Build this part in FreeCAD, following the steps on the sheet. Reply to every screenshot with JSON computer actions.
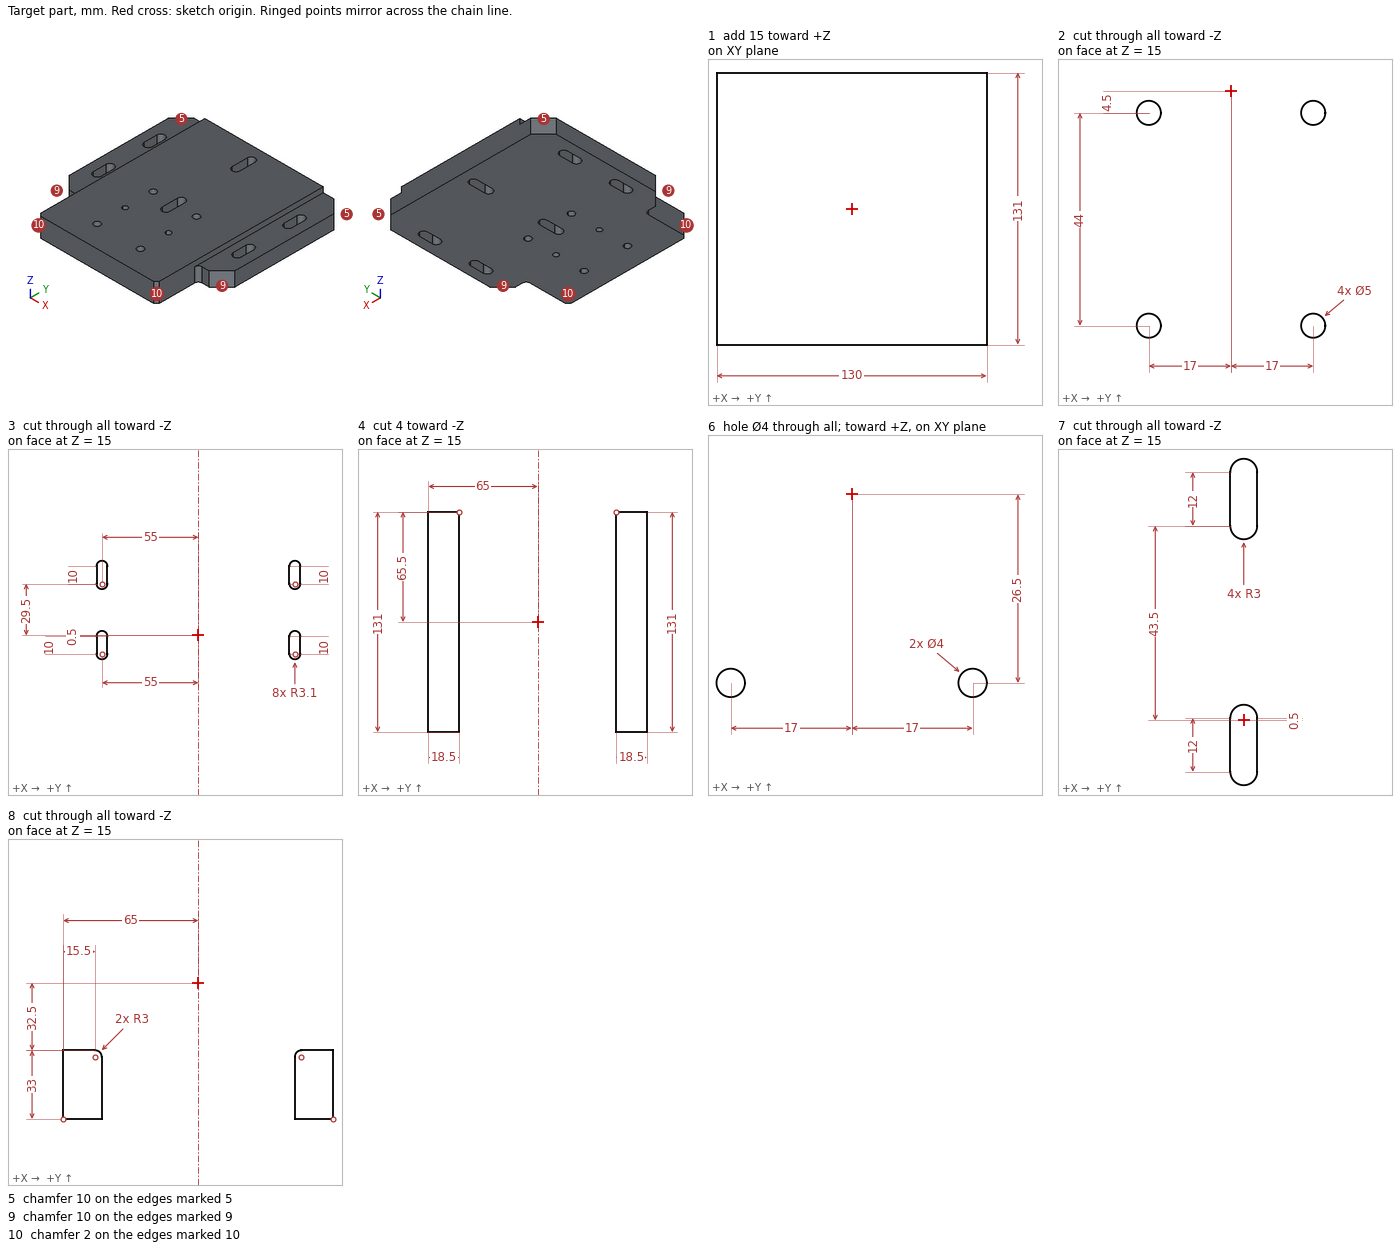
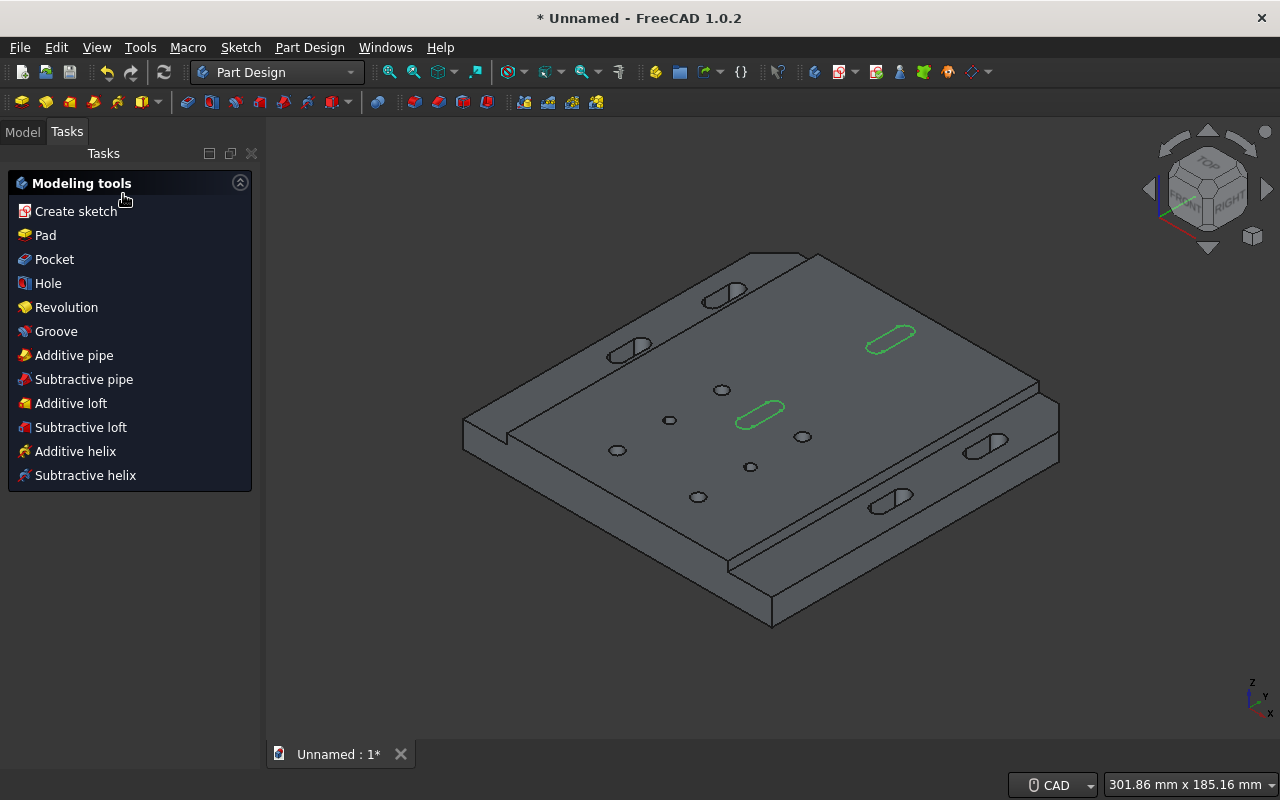
{"action": "left_click", "coordinate": [188, 102]}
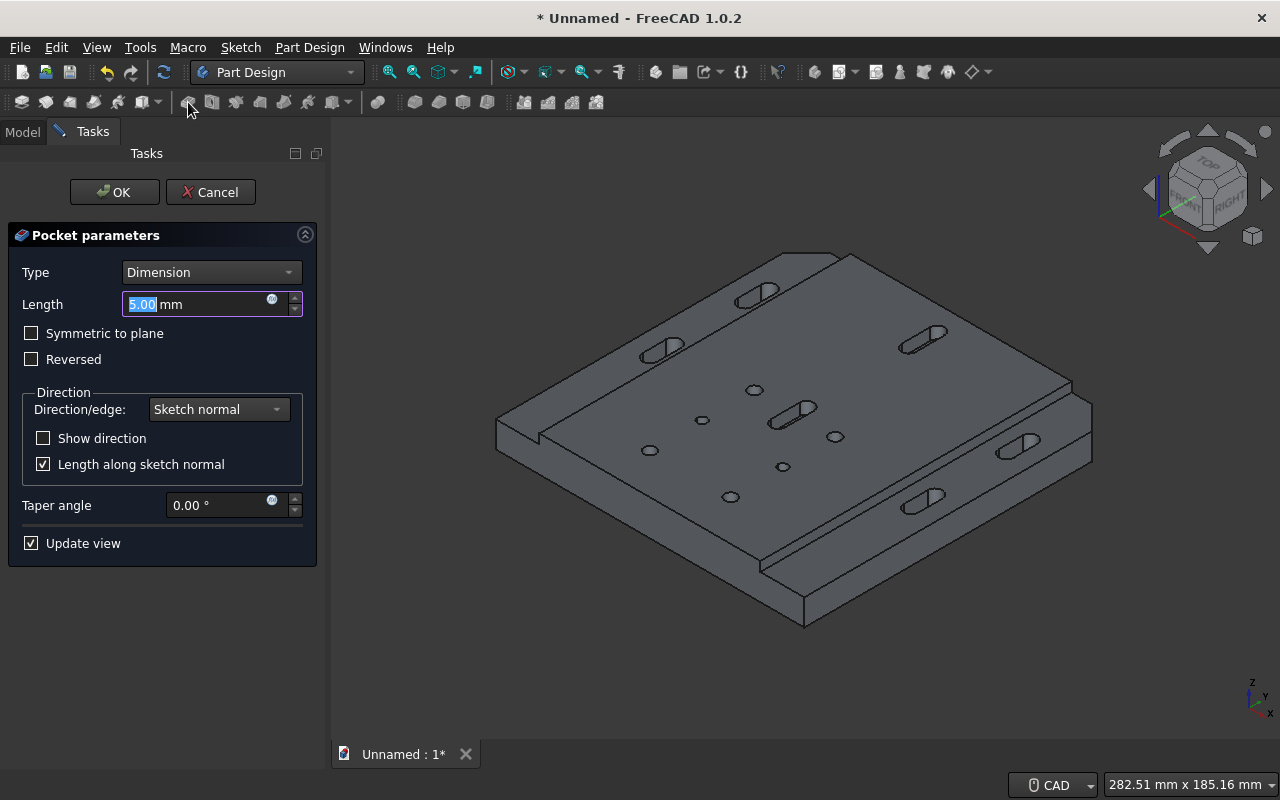
{"action": "left_click", "coordinate": [212, 272]}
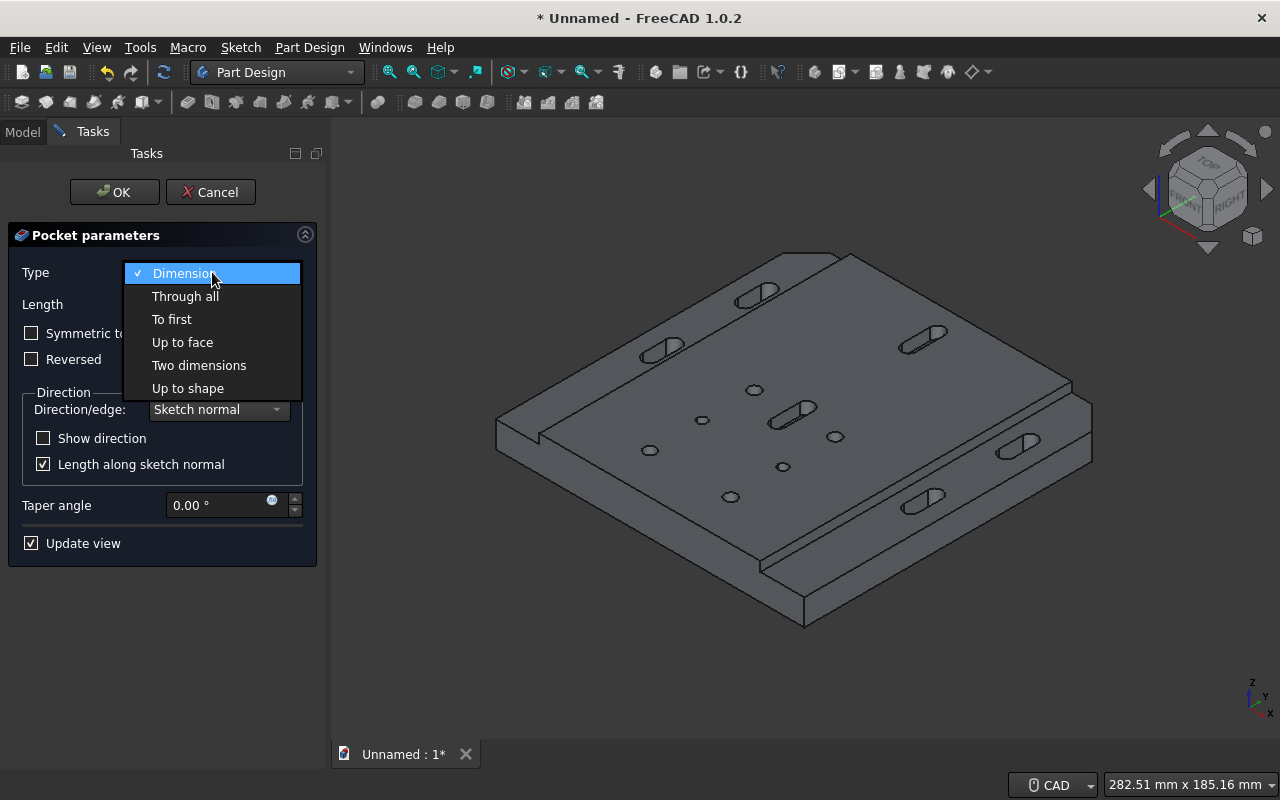
{"action": "left_click", "coordinate": [212, 296]}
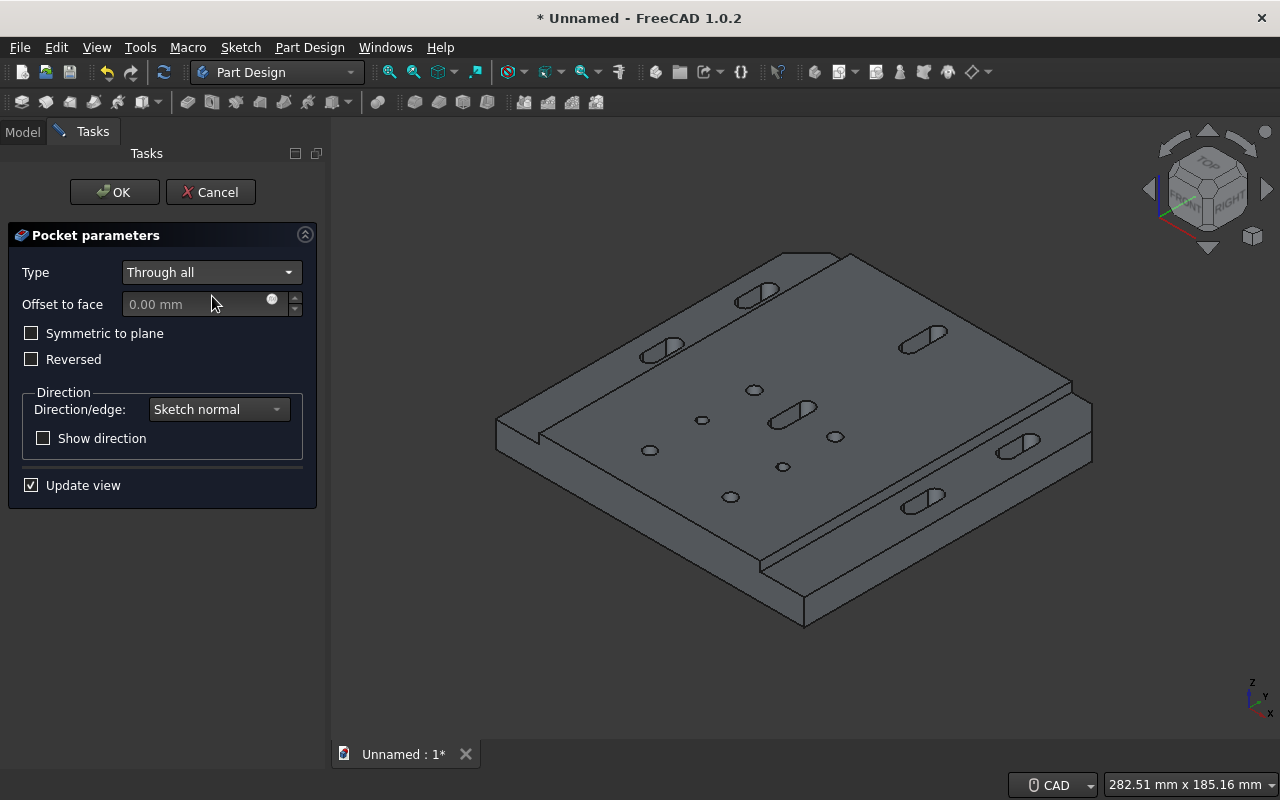
{"action": "left_click", "coordinate": [115, 192]}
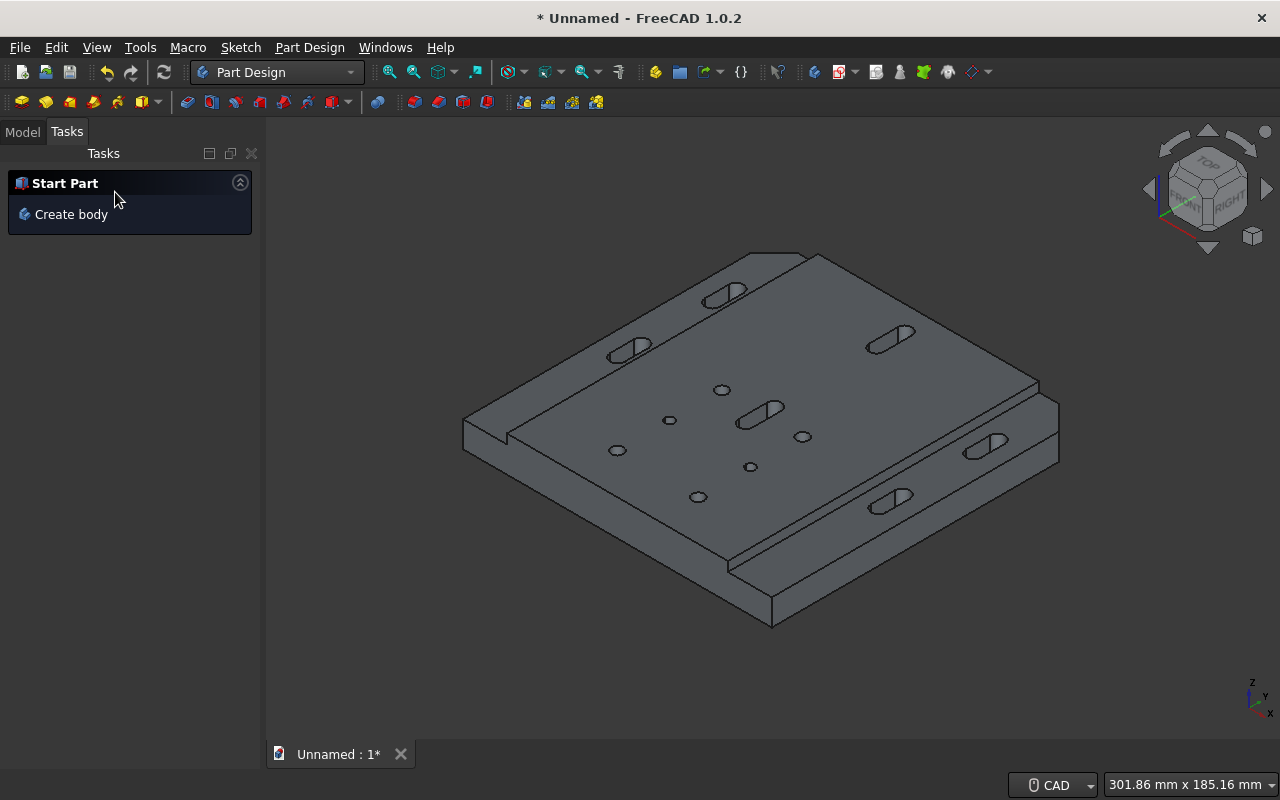
{"action": "left_click", "coordinate": [925, 392]}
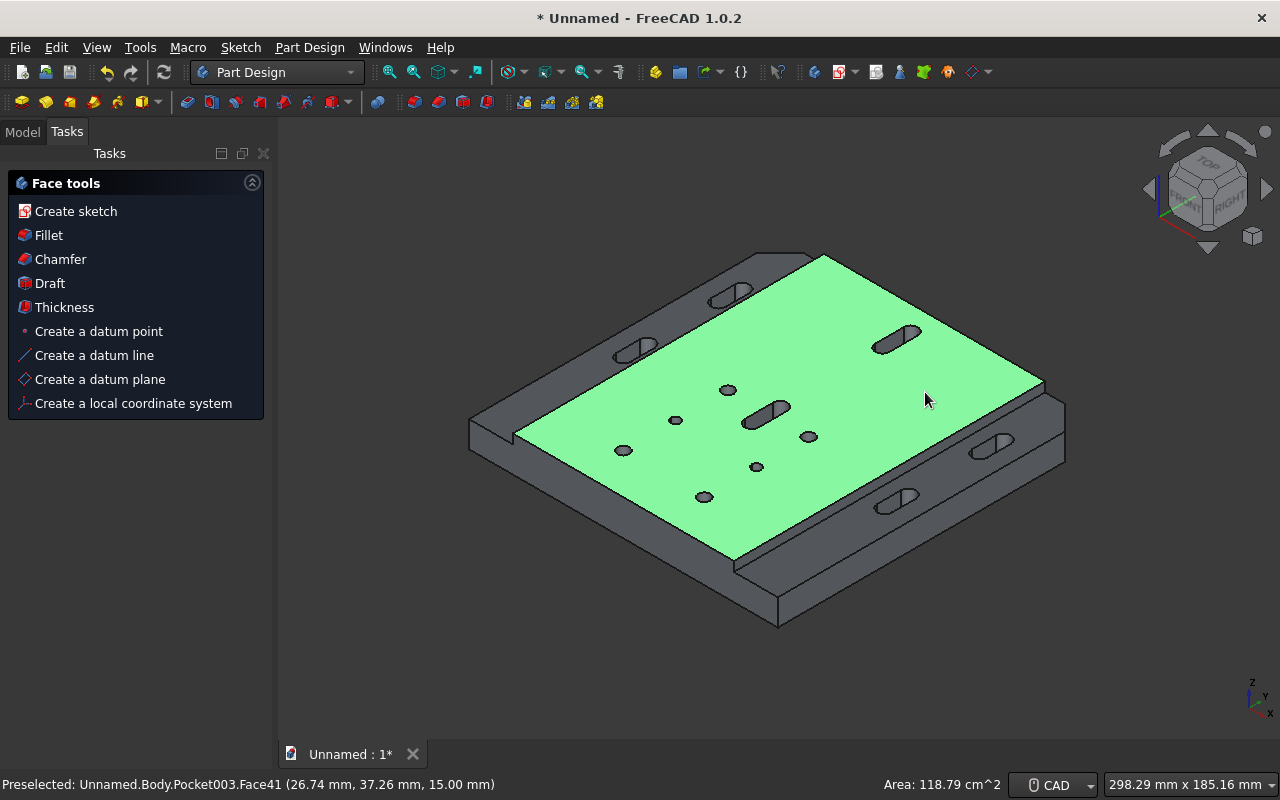
{"action": "left_click", "coordinate": [840, 72]}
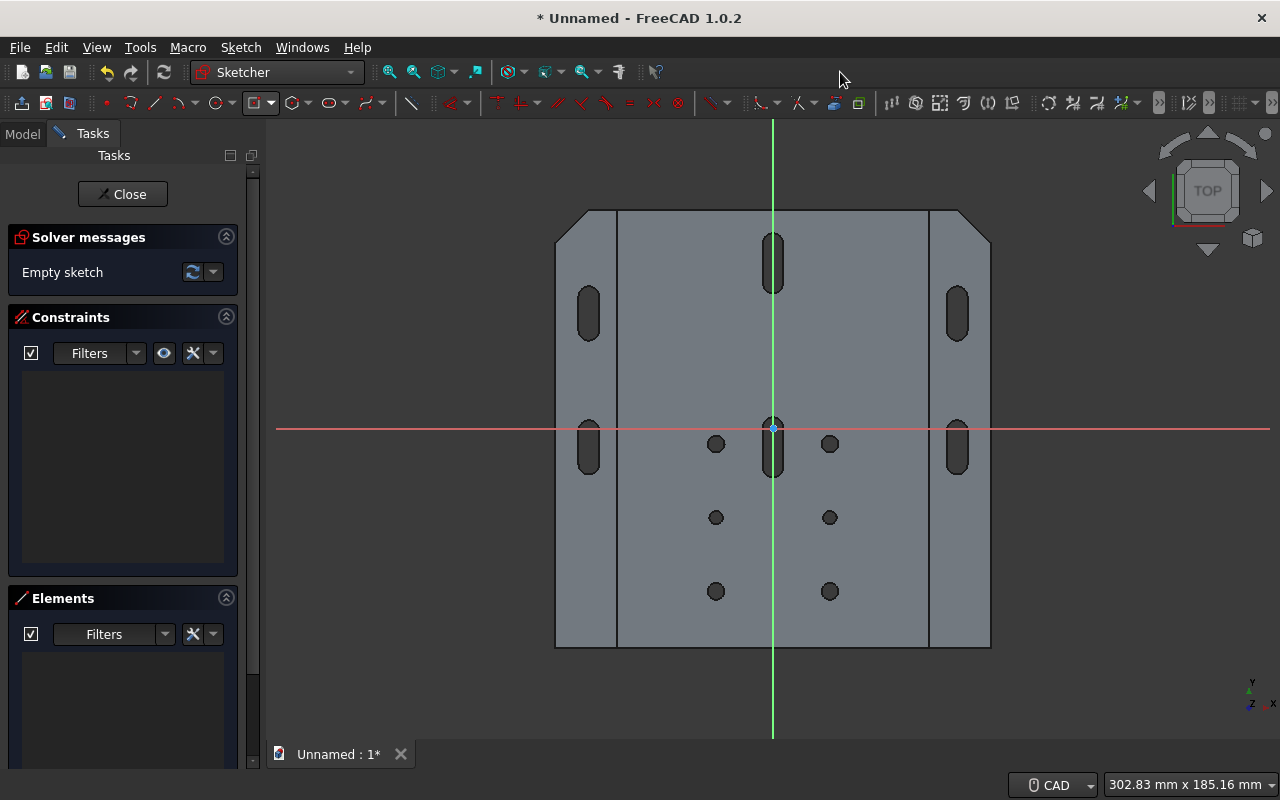
{"action": "left_click", "coordinate": [132, 104]}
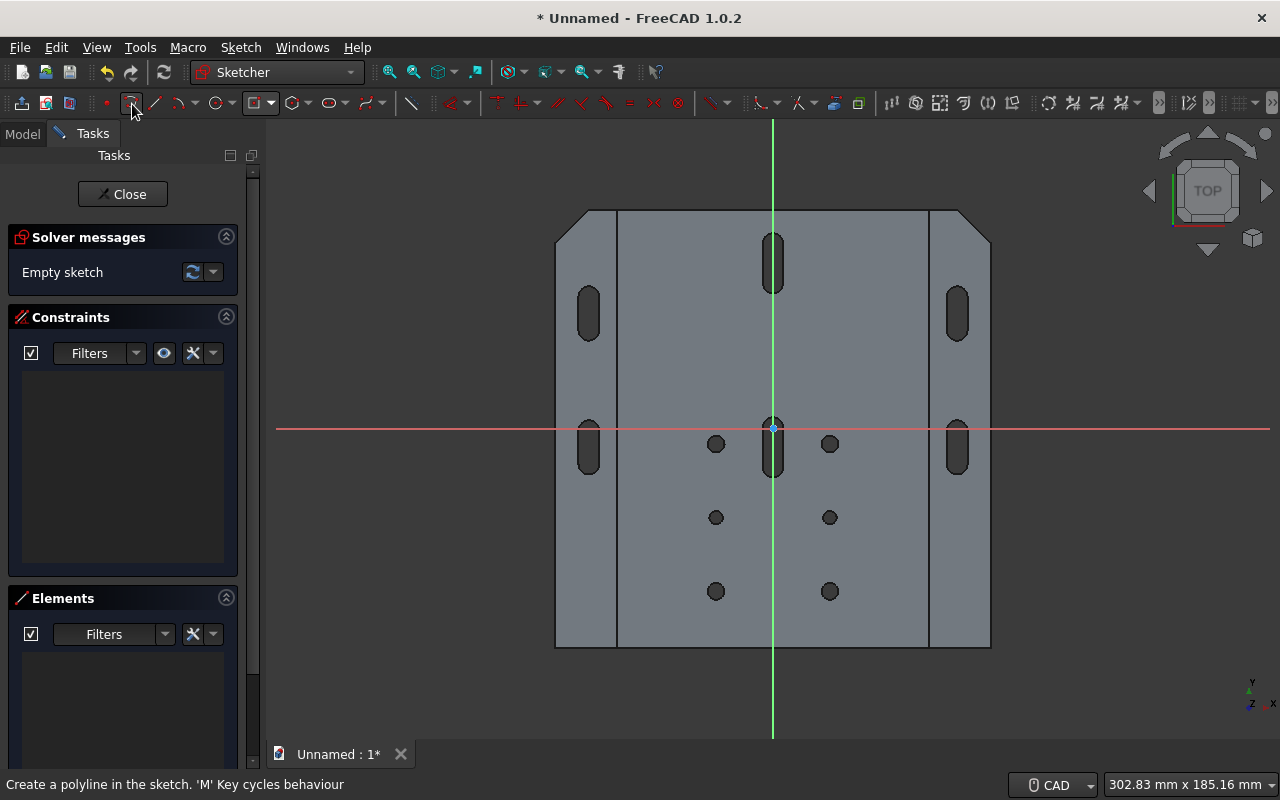
{"action": "left_click", "coordinate": [607, 538]}
{"action": "left_click", "coordinate": [555, 538]}
{"action": "left_click", "coordinate": [555, 648]}
{"action": "left_click", "coordinate": [617, 648]}
{"action": "left_click", "coordinate": [617, 548]}
{"action": "right_click", "coordinate": [617, 548]}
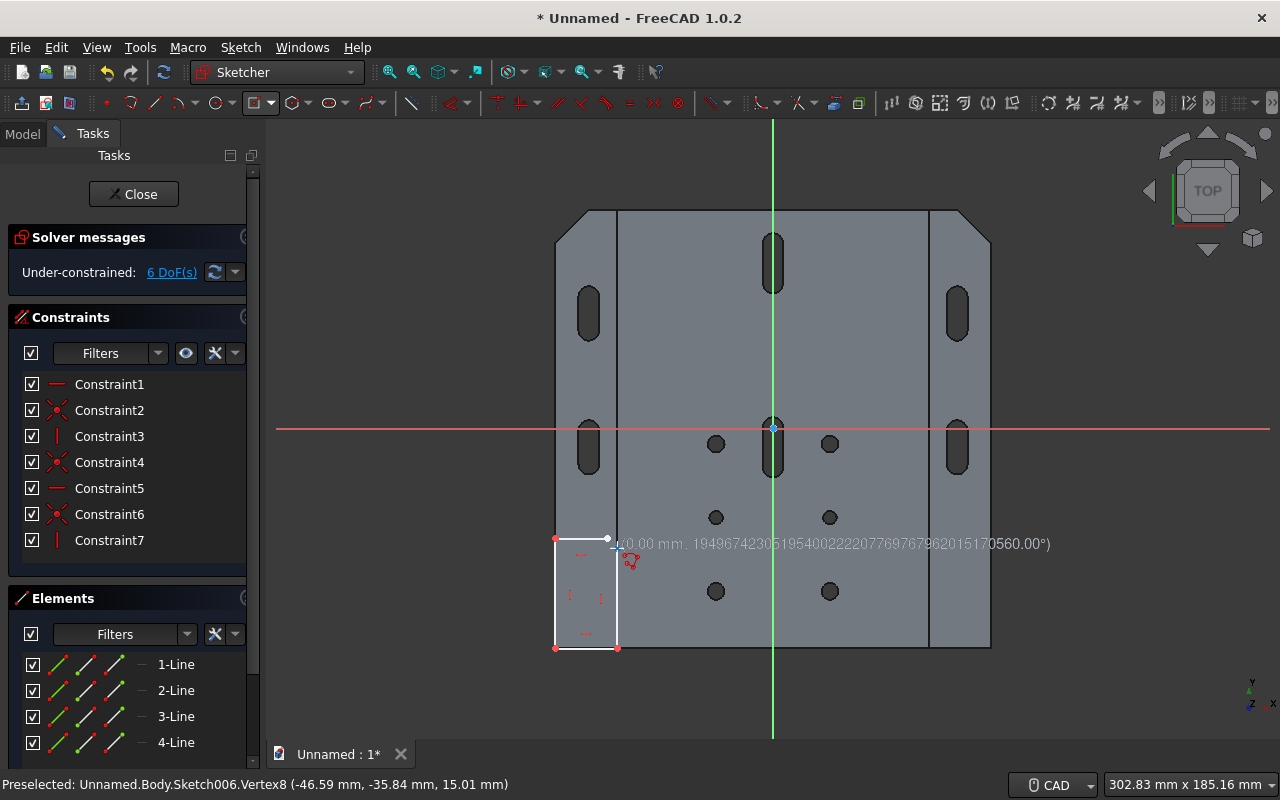
{"action": "left_click", "coordinate": [198, 104]}